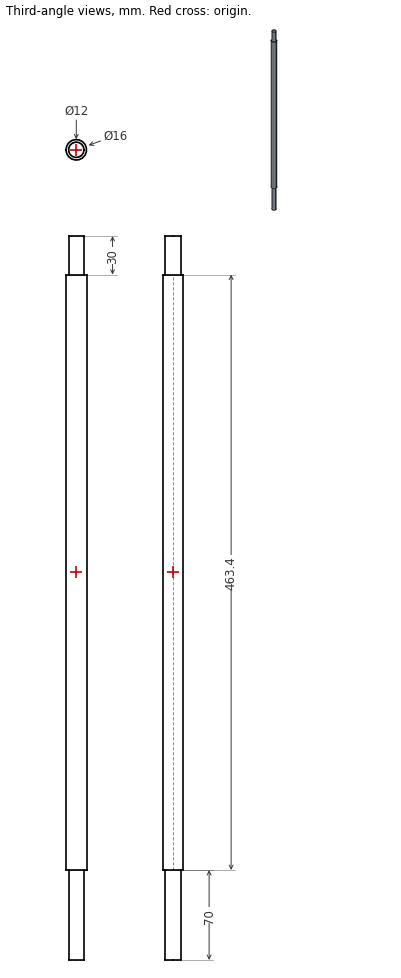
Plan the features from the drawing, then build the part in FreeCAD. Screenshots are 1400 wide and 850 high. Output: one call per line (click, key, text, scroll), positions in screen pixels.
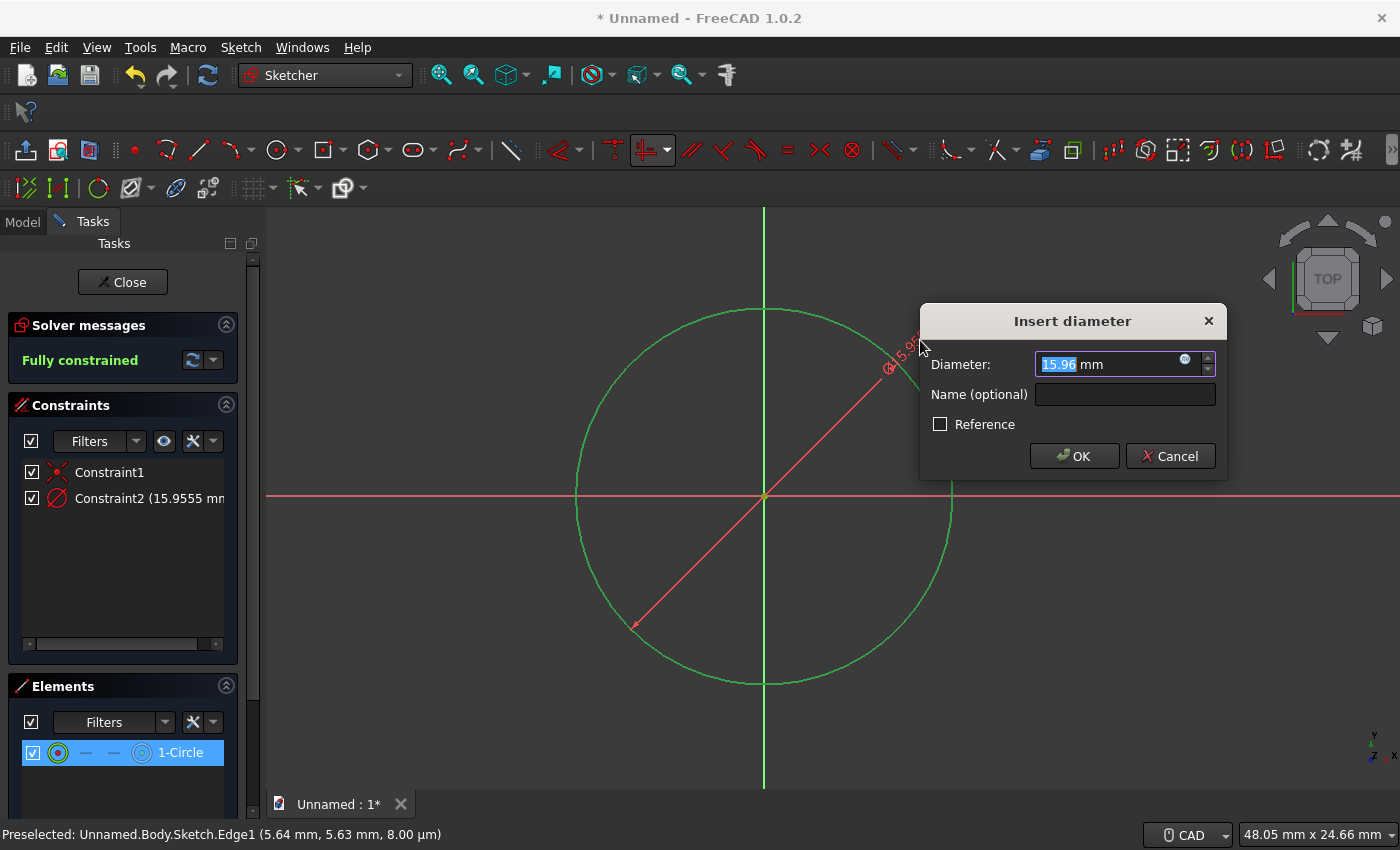
text(16)
key(Return)
key(Escape)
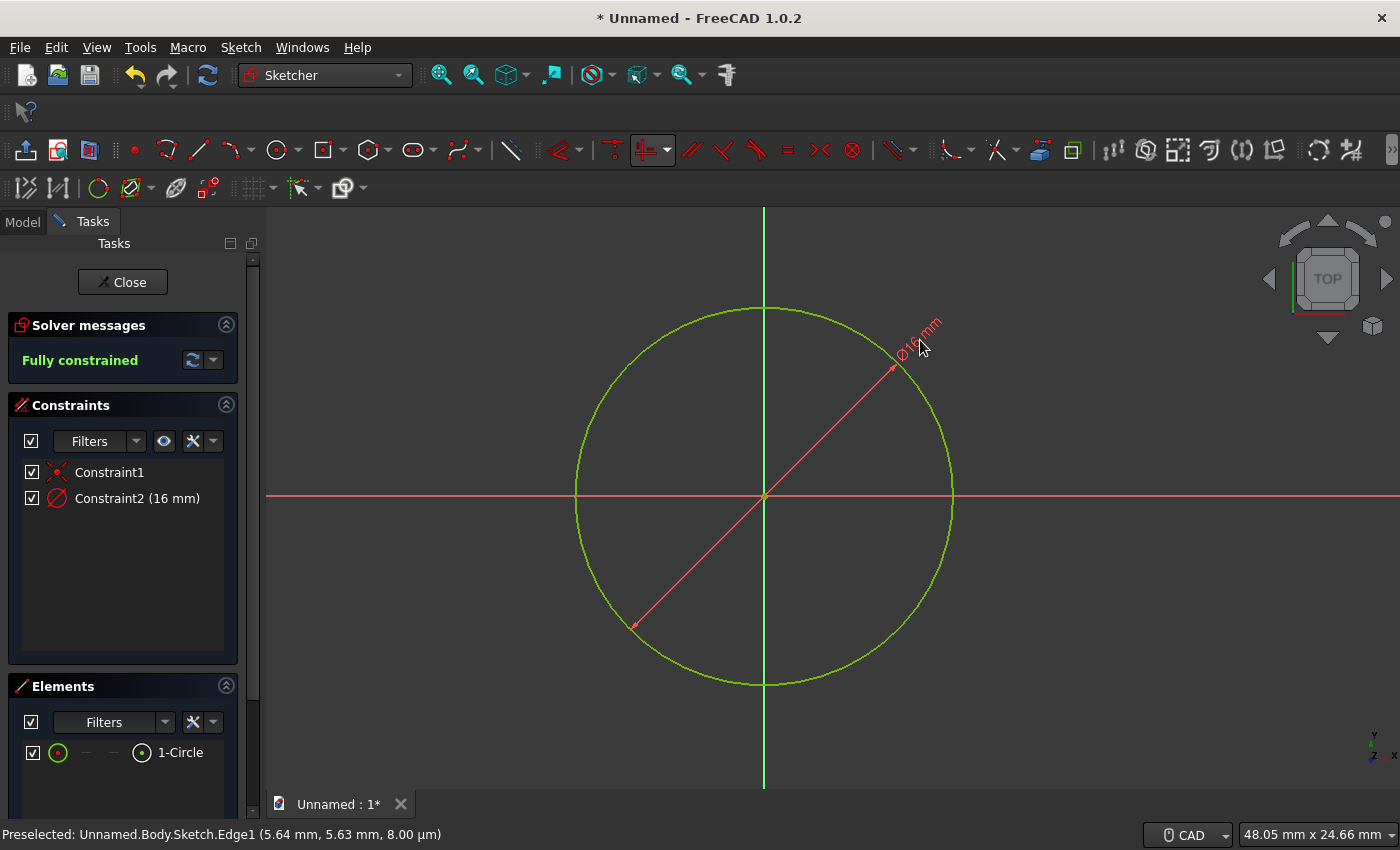
click(123, 282)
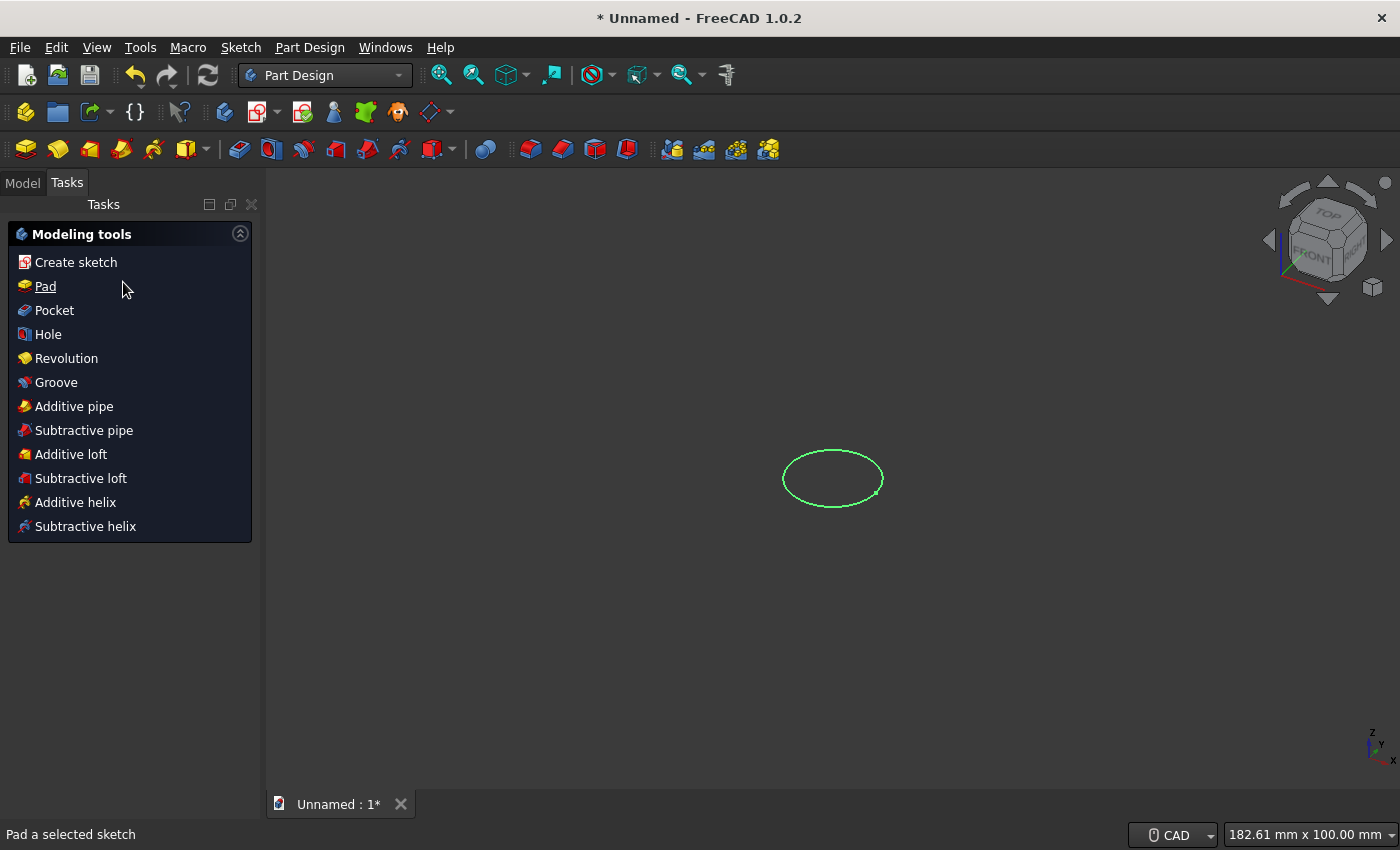
click(26, 150)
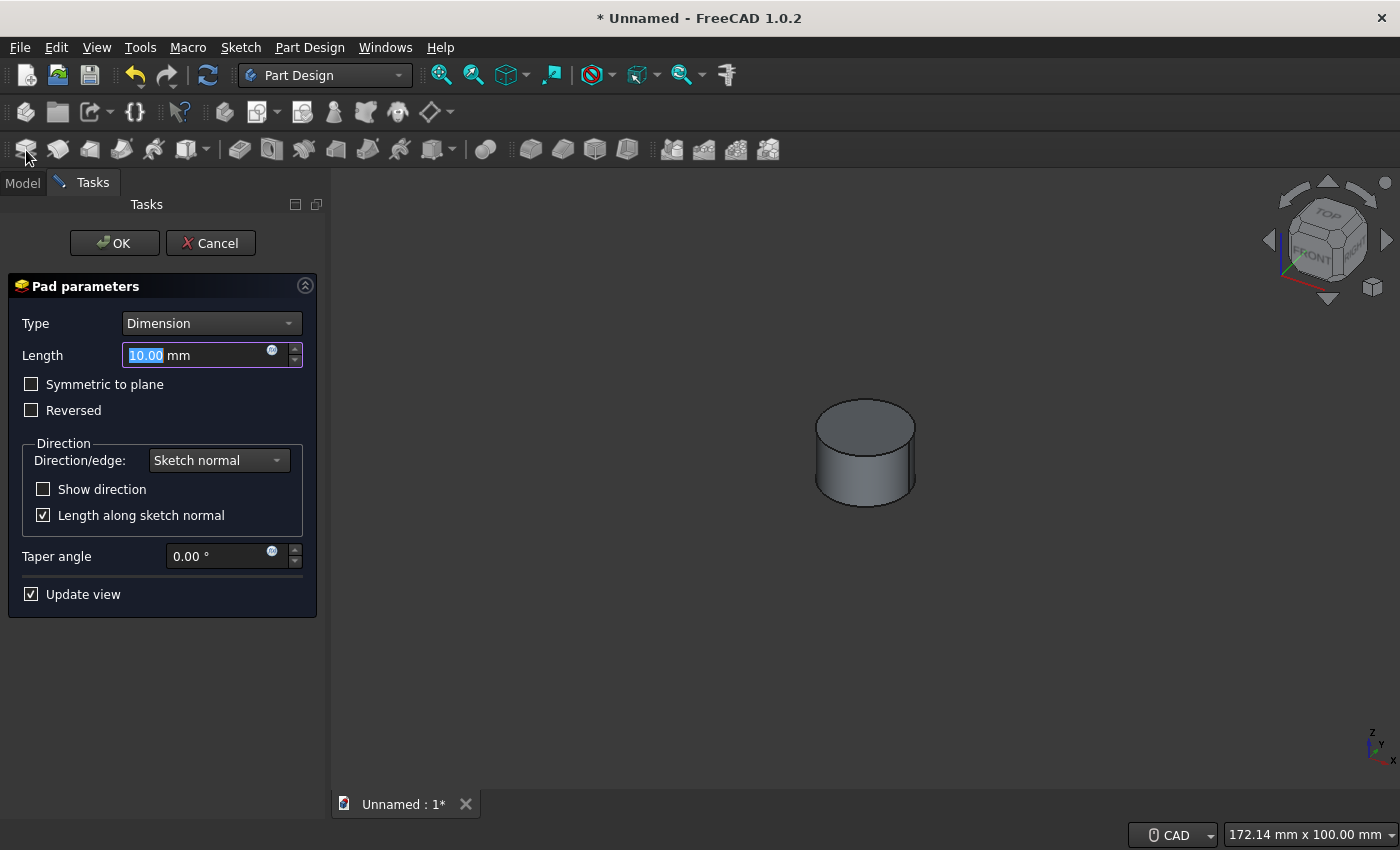
text(463.4)
key(Tab)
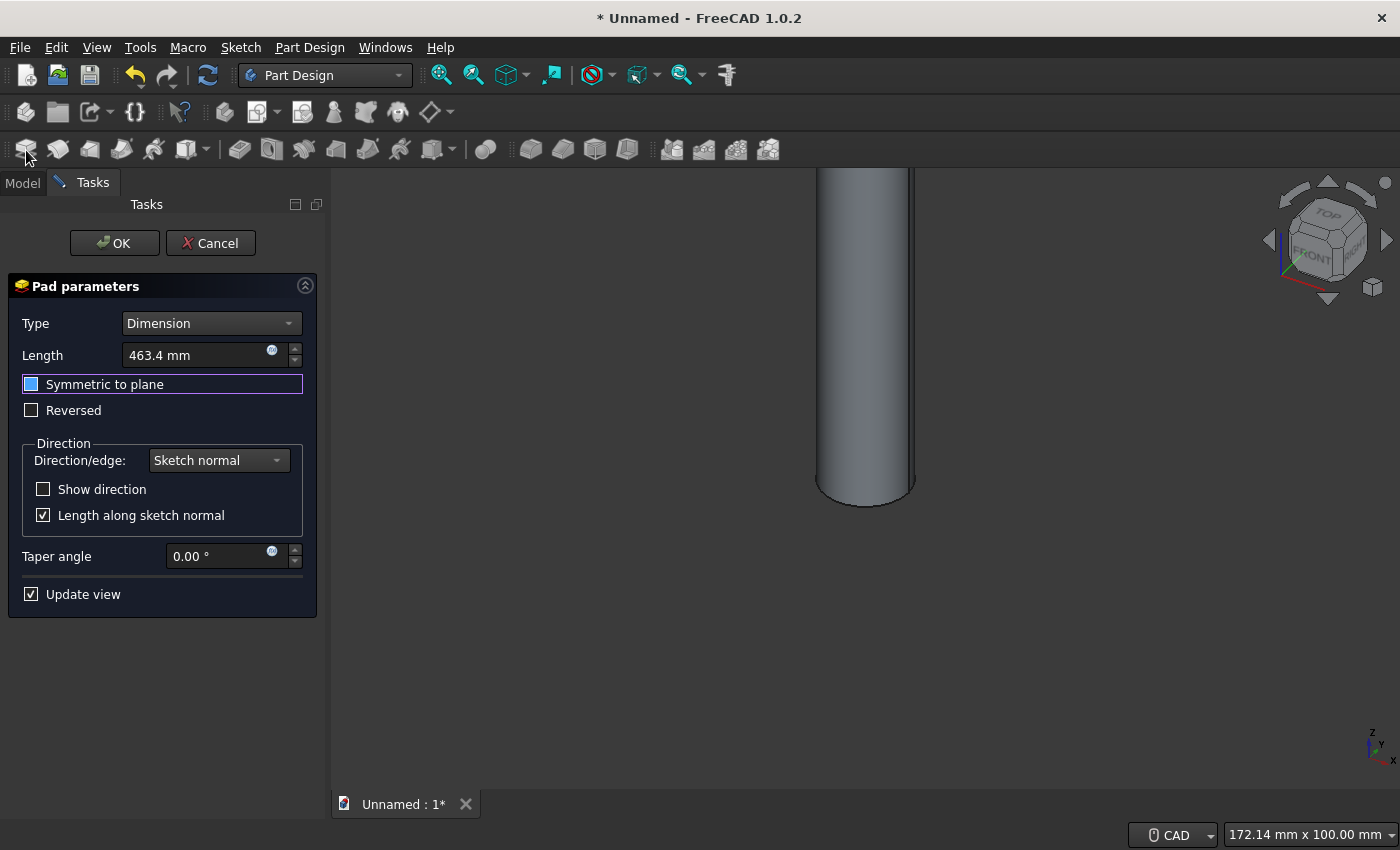
click(30, 384)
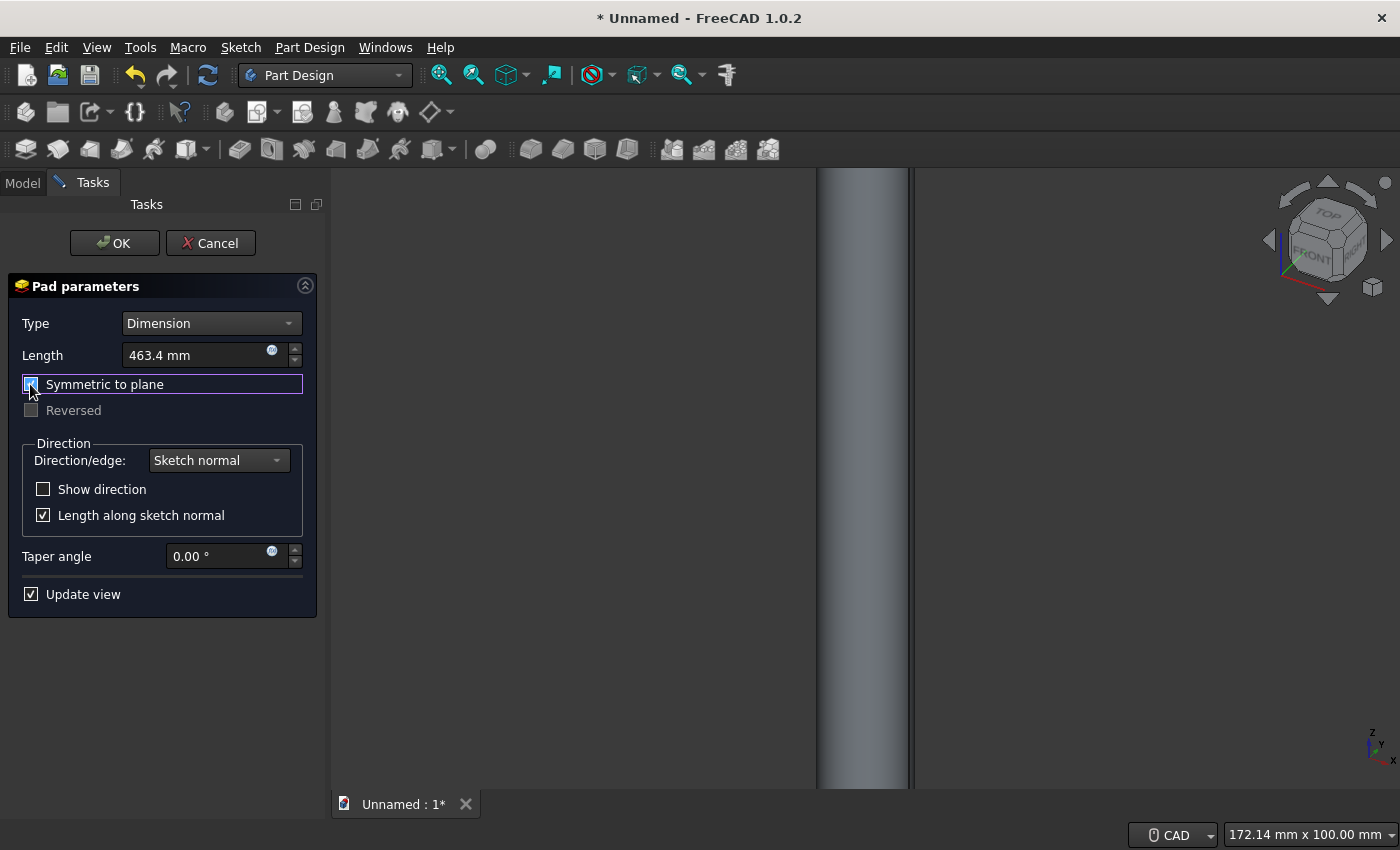
click(115, 243)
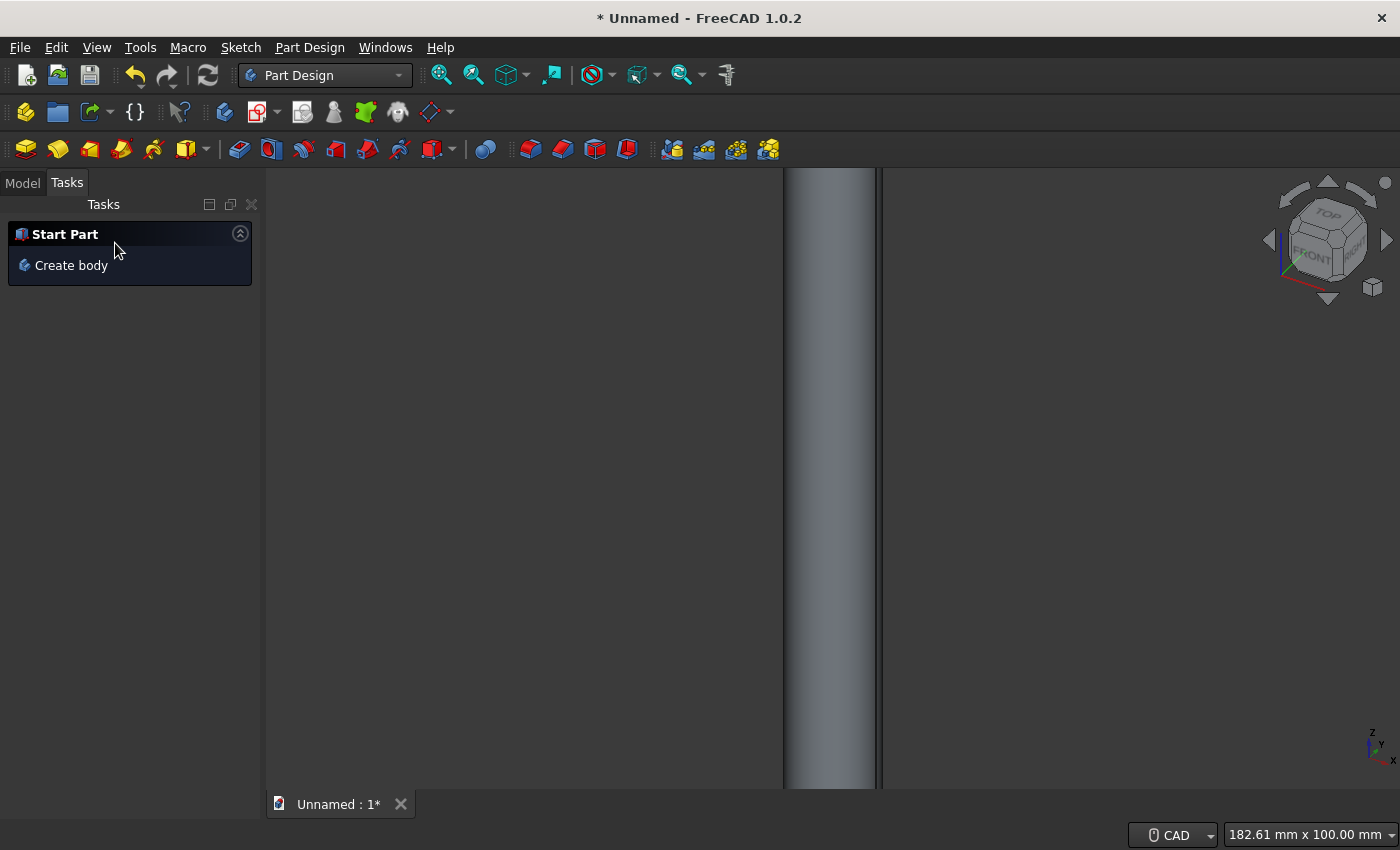
key(v)
key(f)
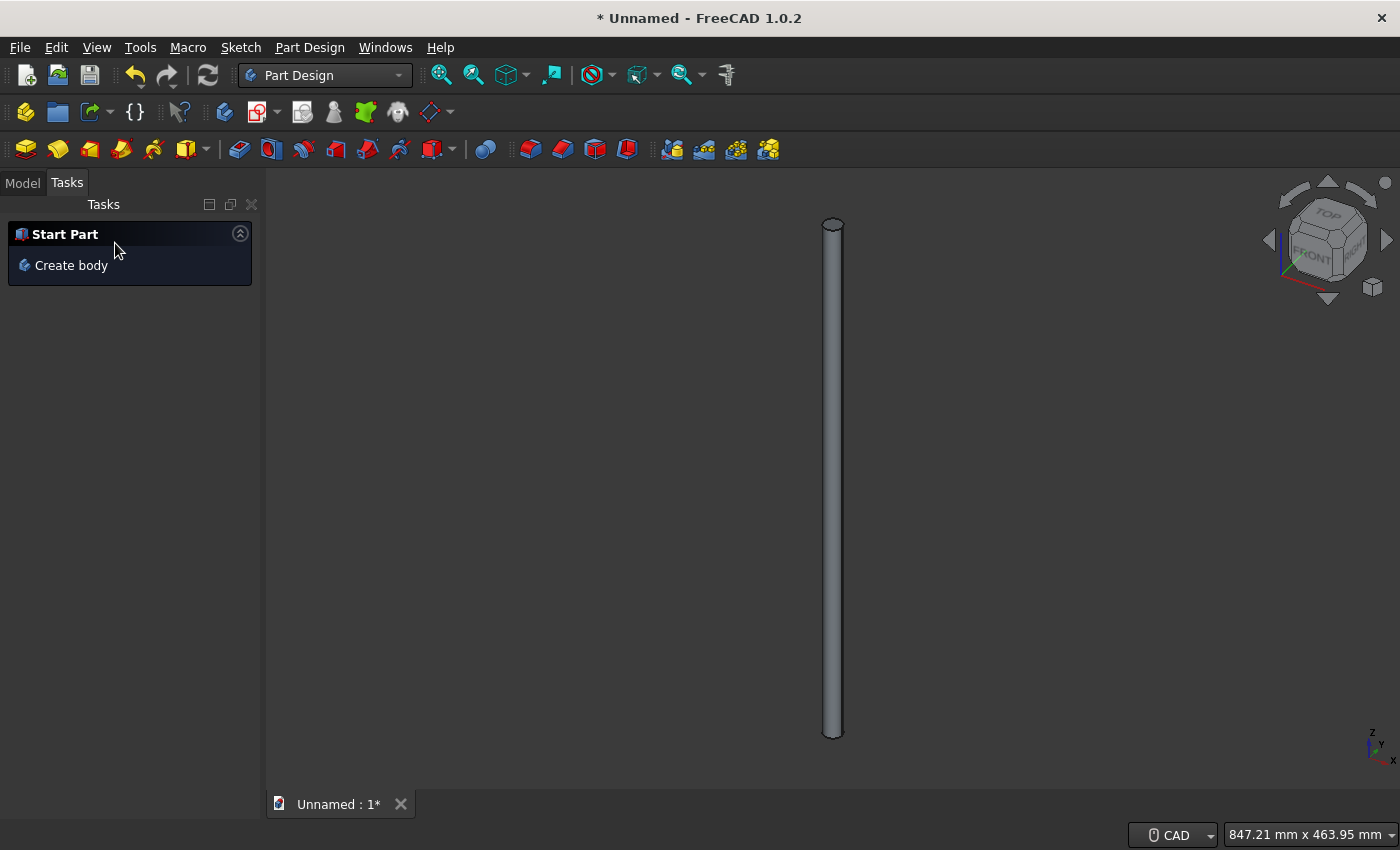
key(0)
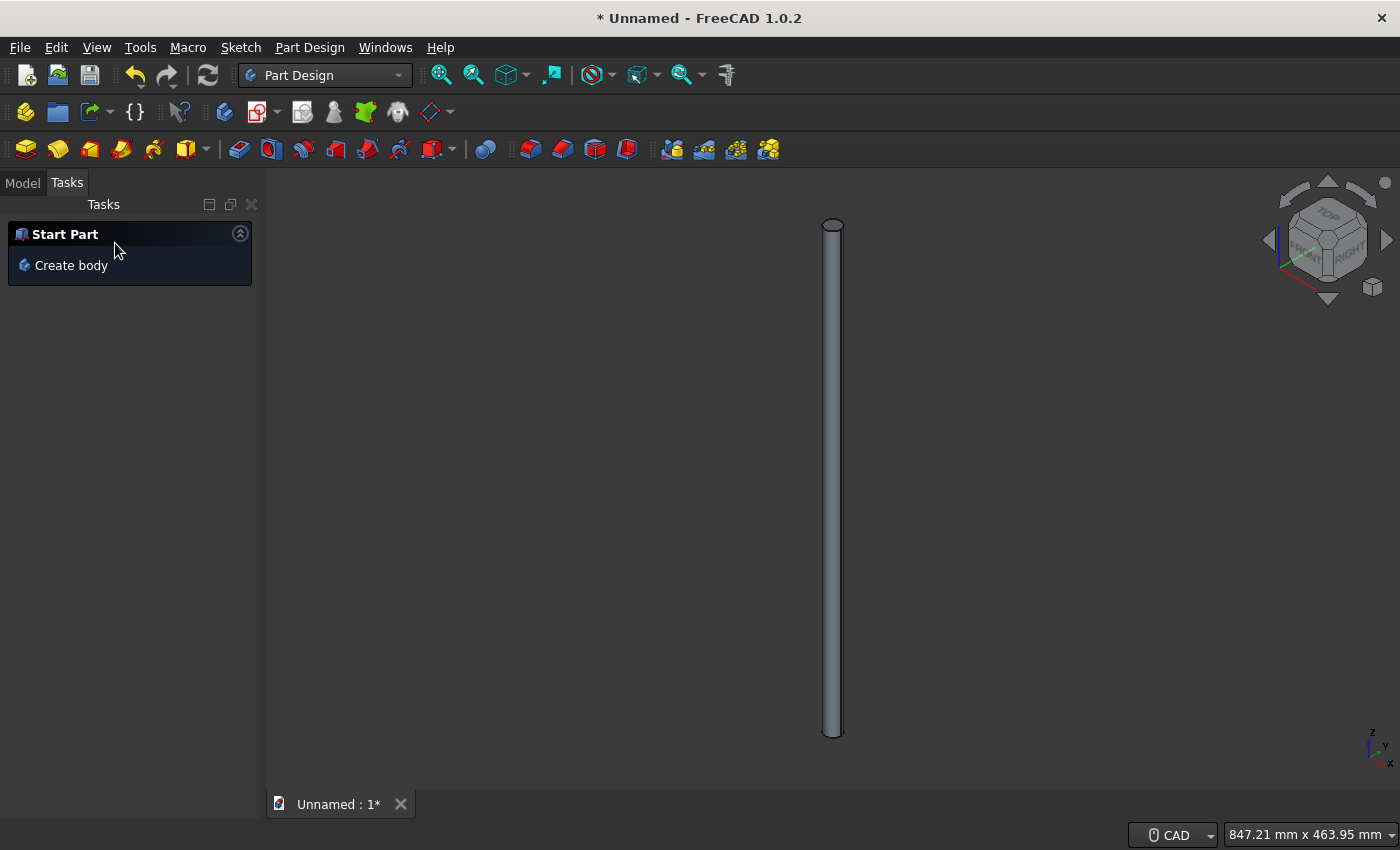
key(2)